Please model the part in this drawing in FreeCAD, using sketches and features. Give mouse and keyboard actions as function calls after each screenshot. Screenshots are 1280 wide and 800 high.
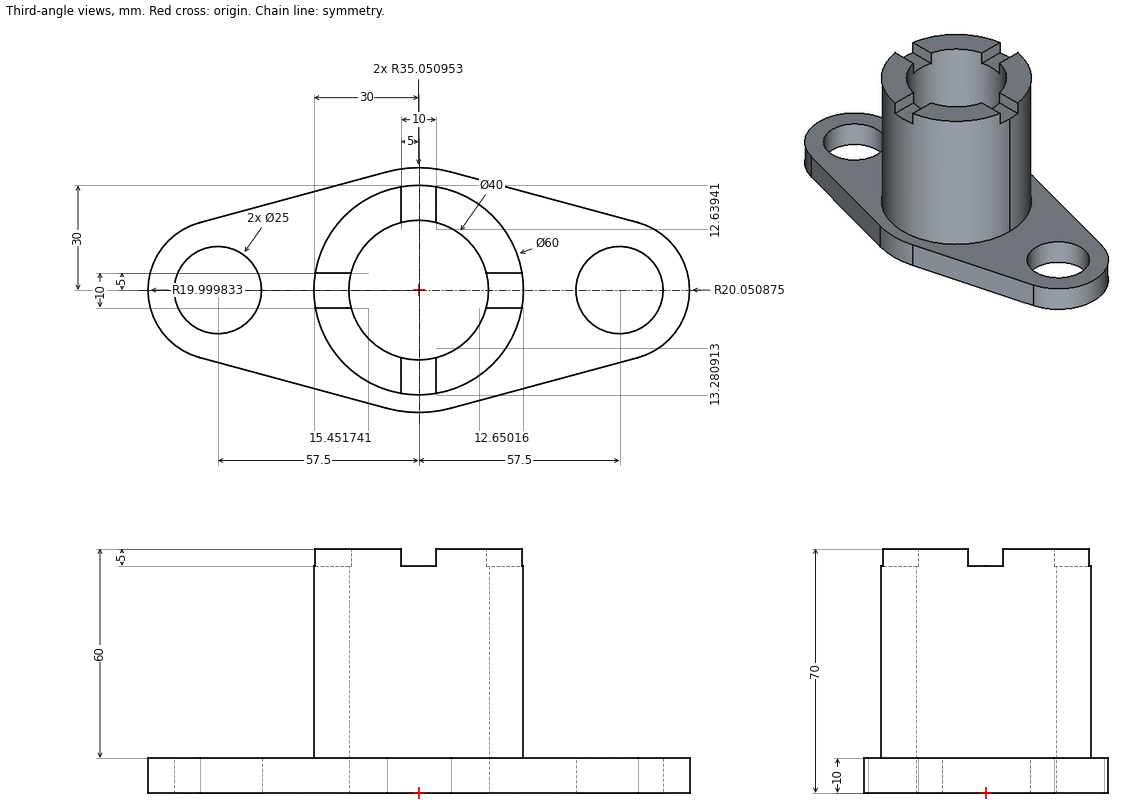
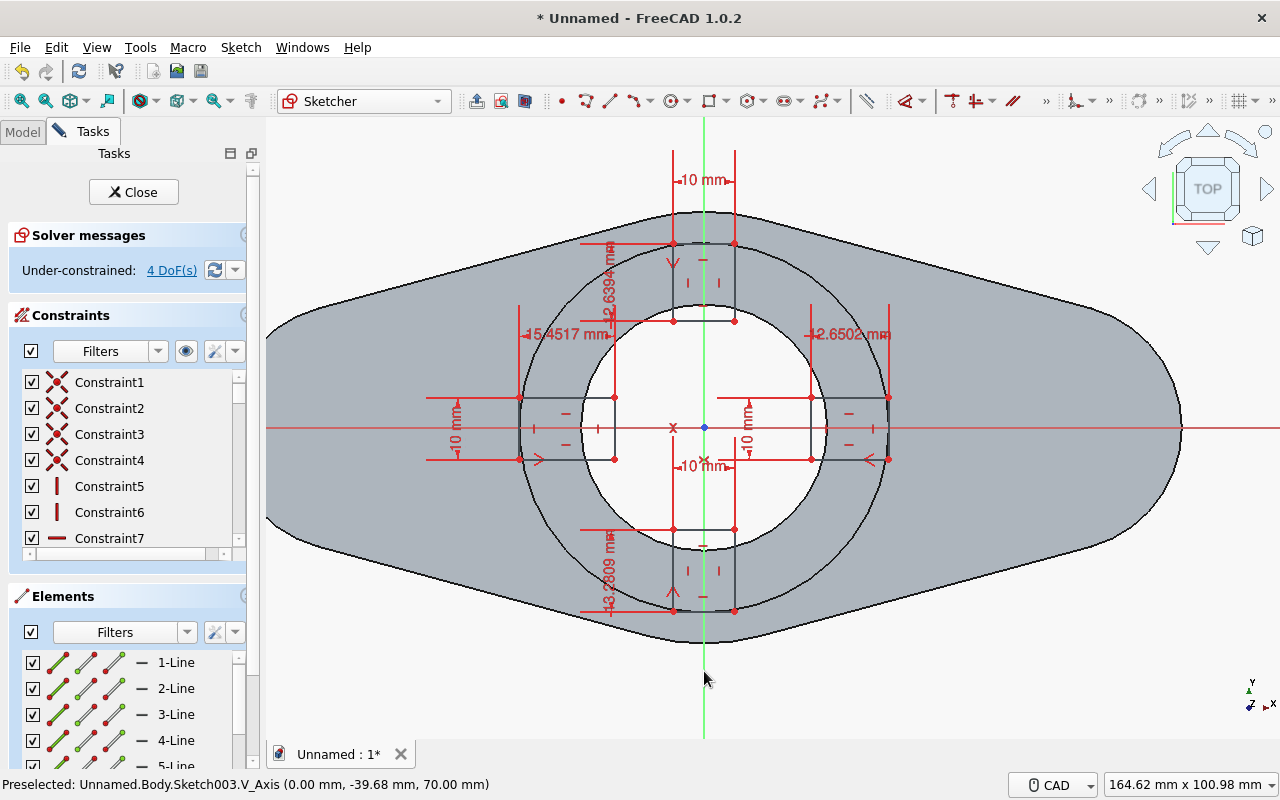
scroll(673, 244, up, 2)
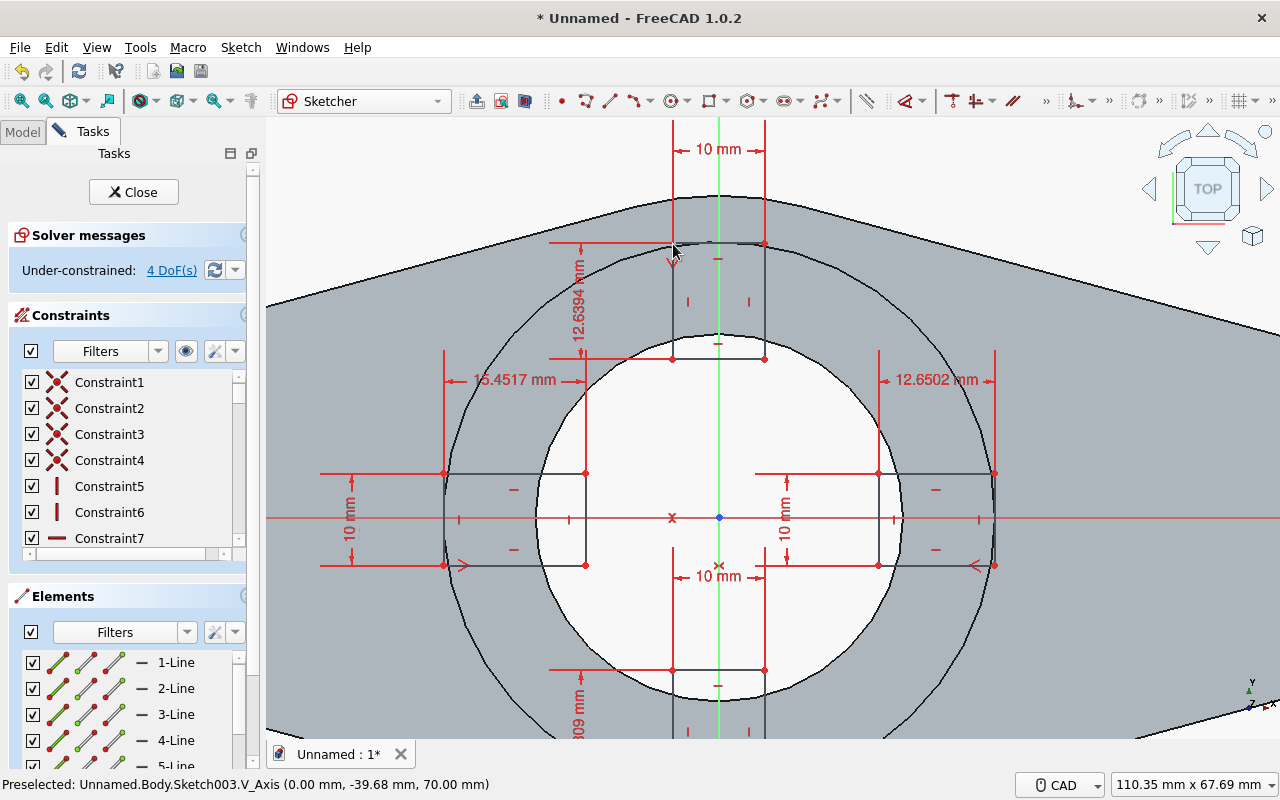
click(673, 243)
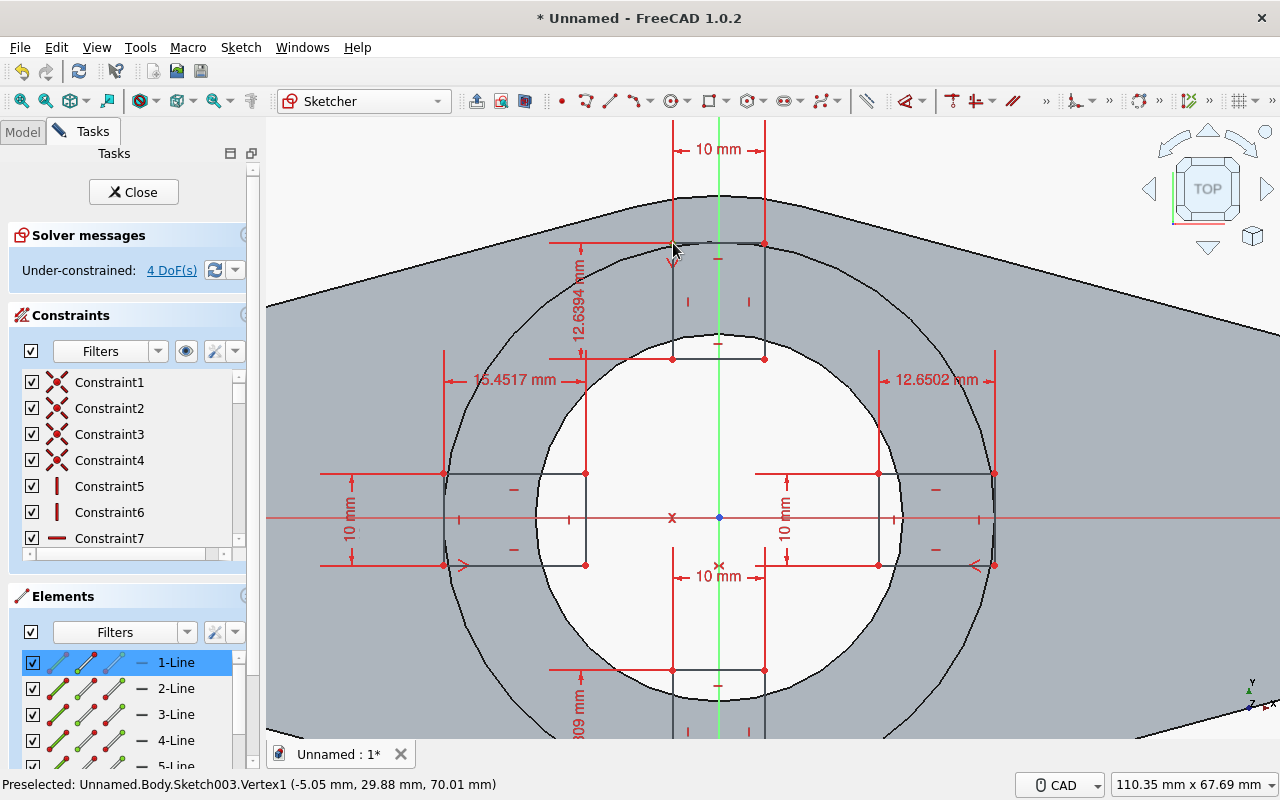
key(l)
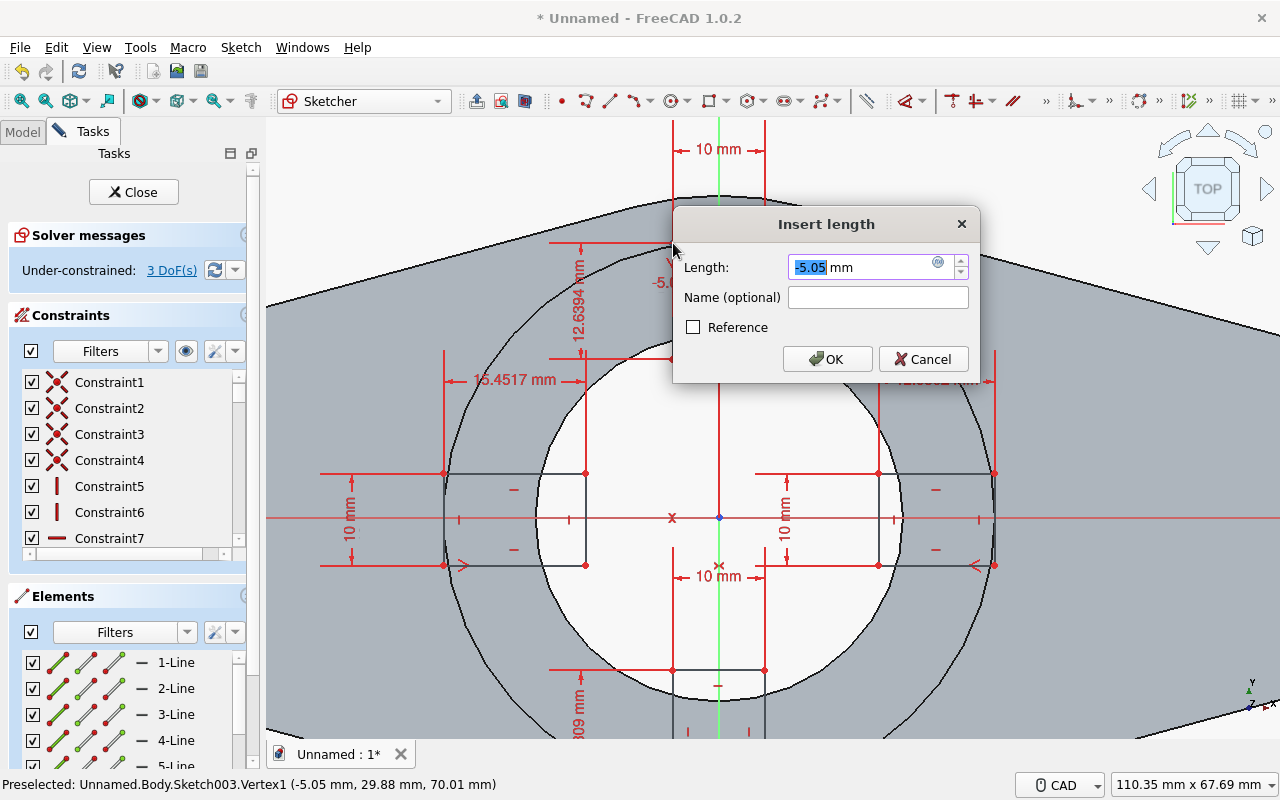
text(-5)
key(Return)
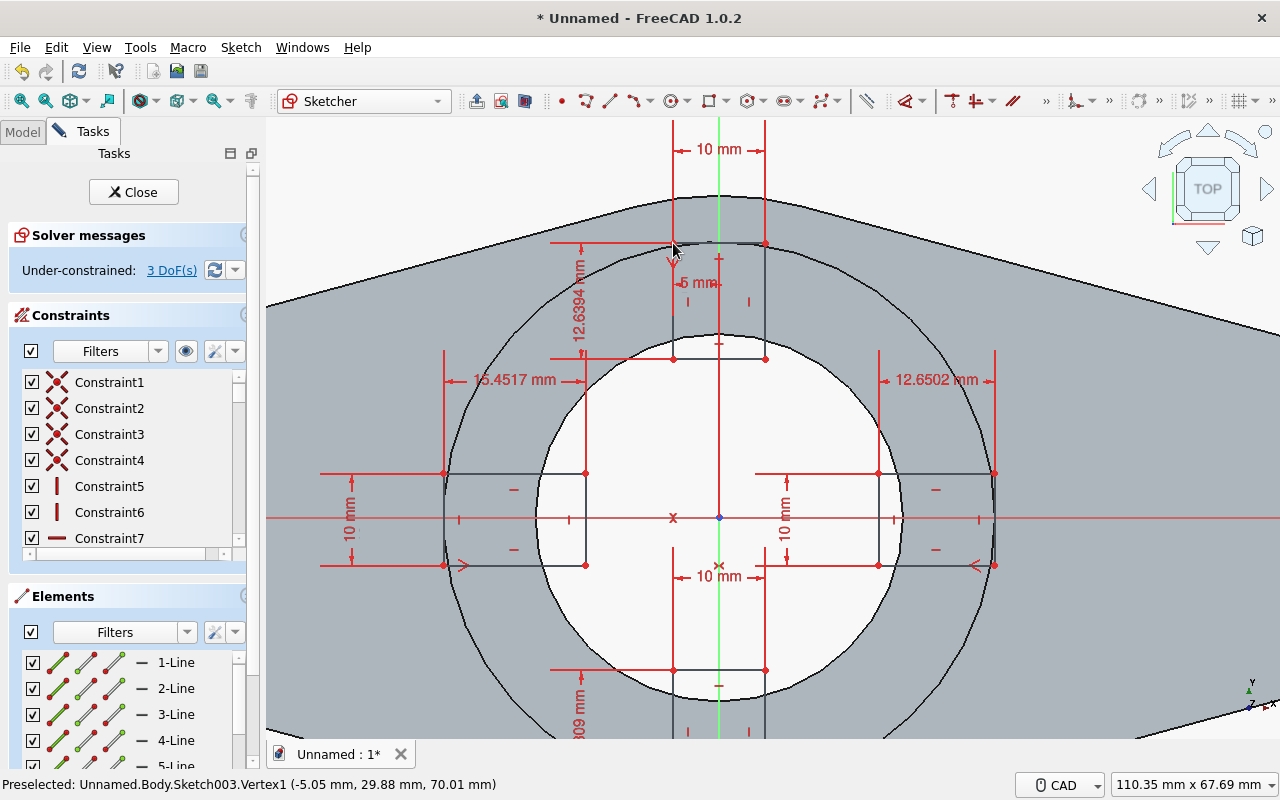
click(444, 474)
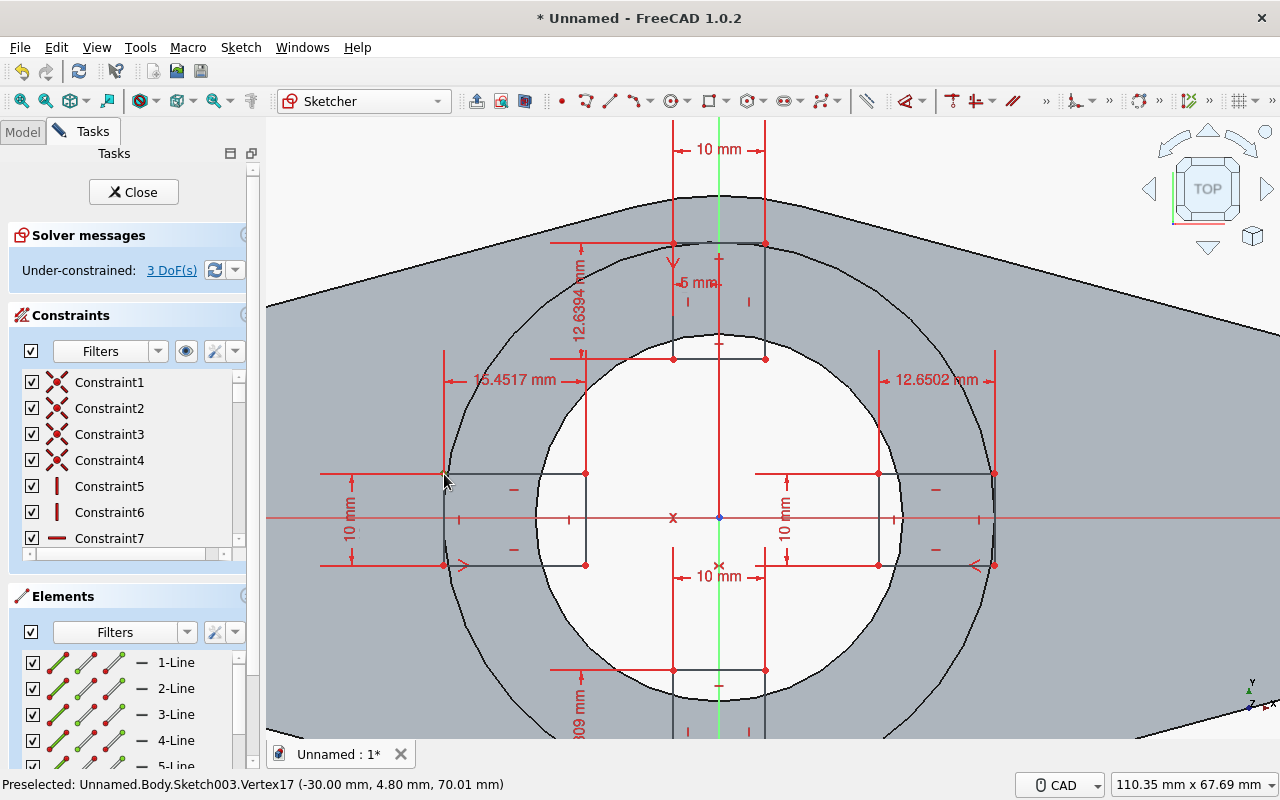
click(924, 102)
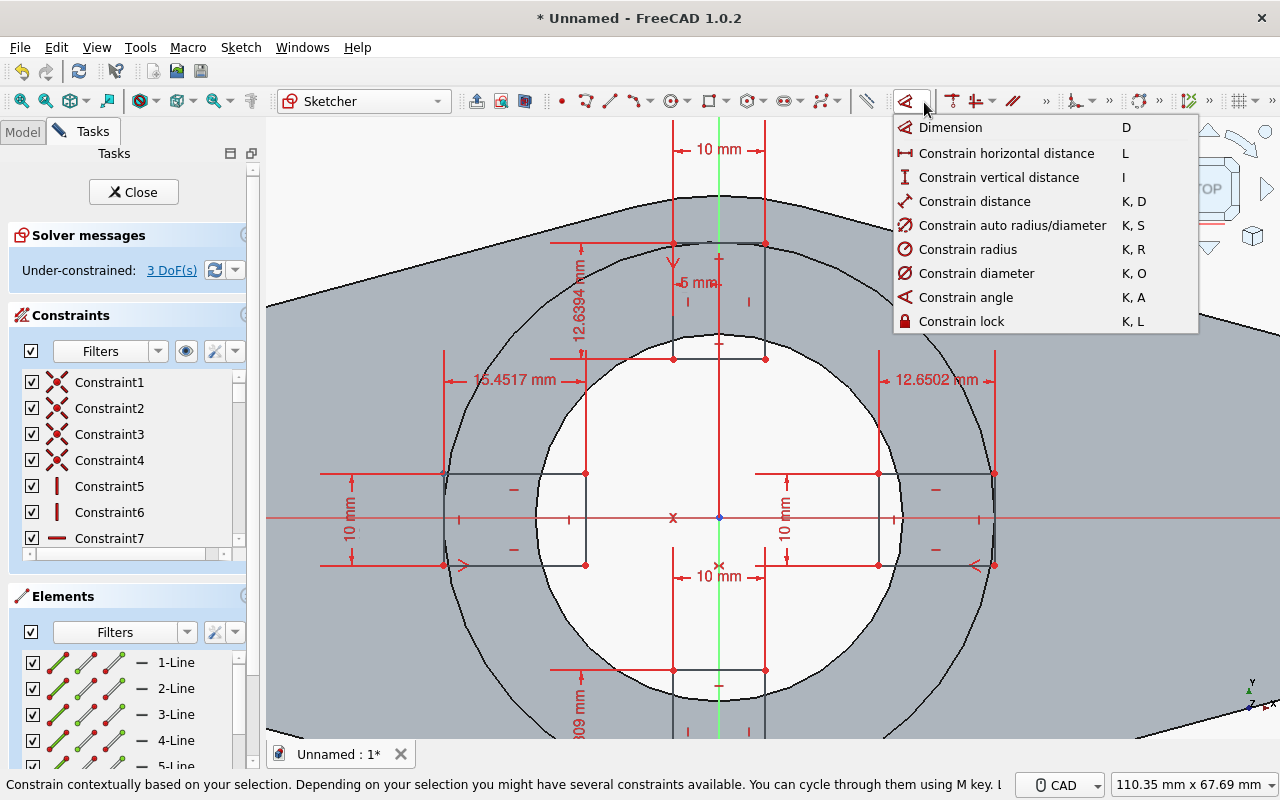
click(1046, 177)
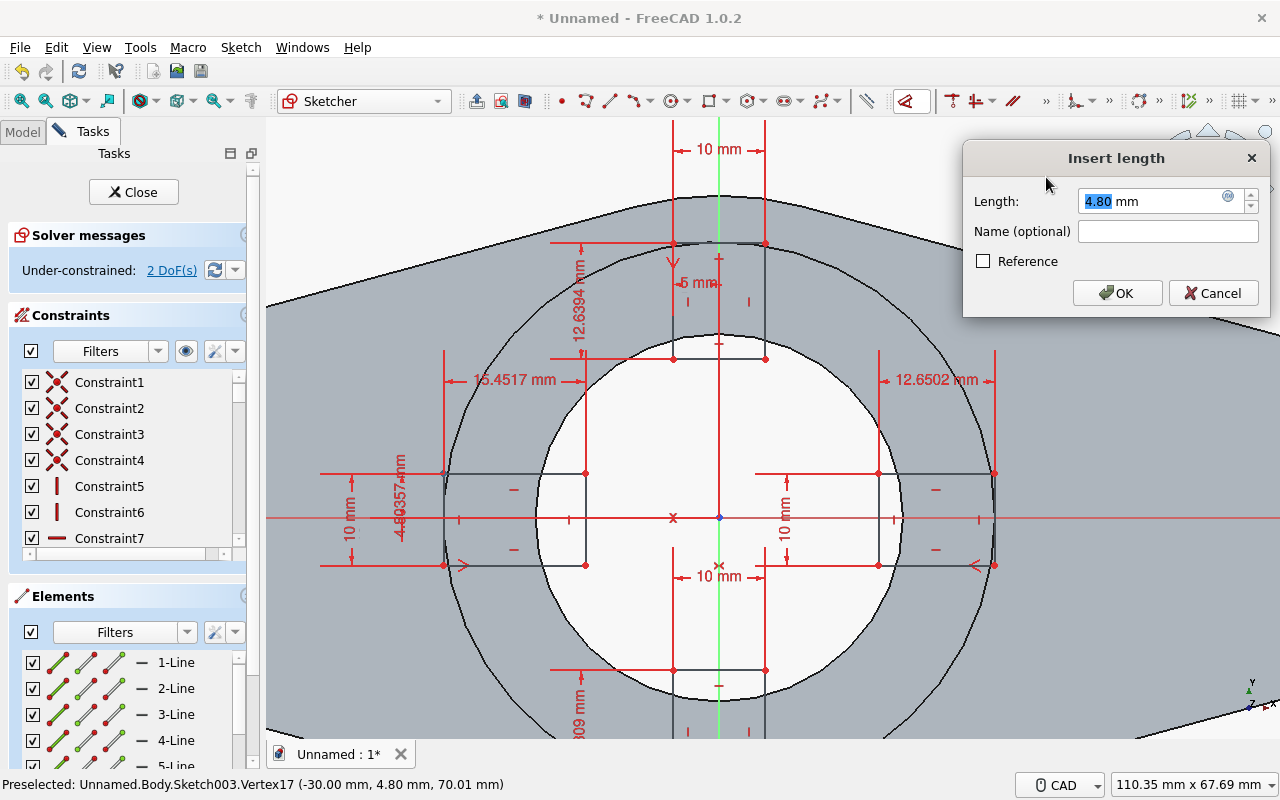
text(5)
key(Return)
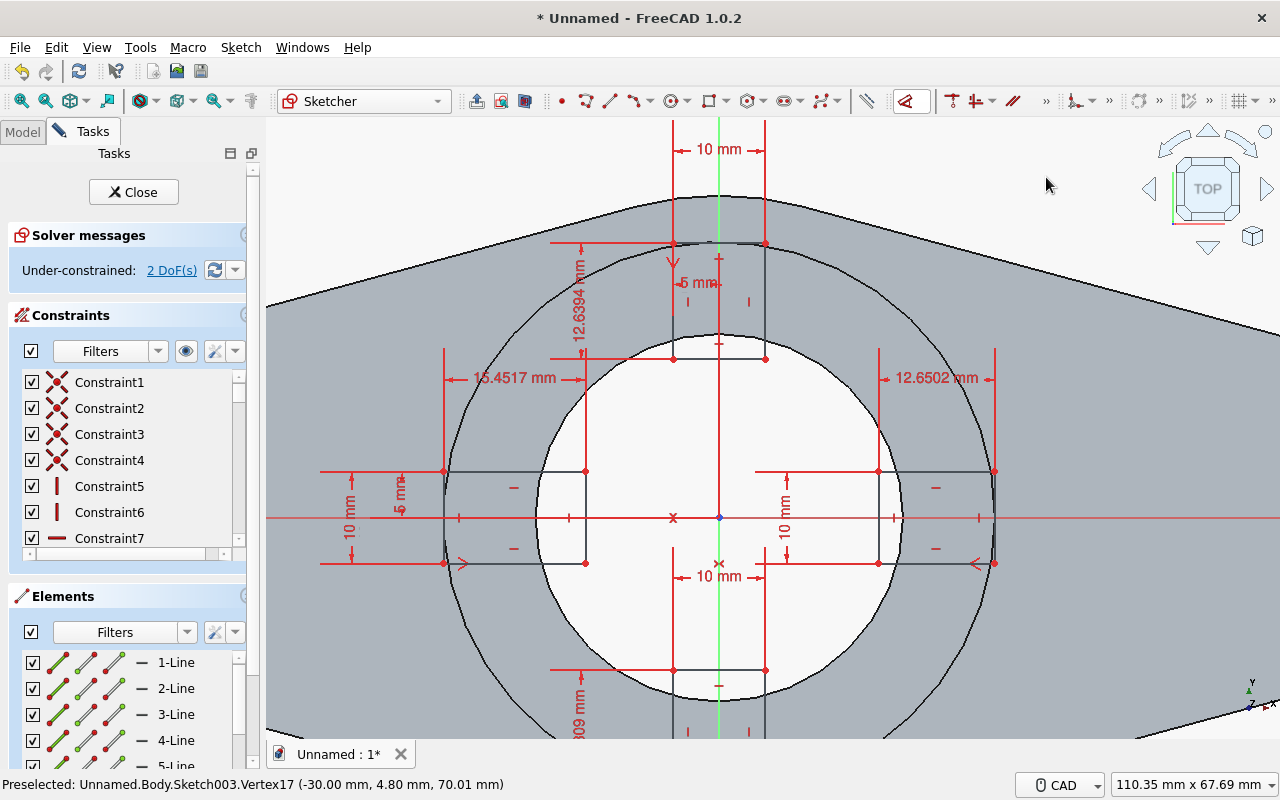
click(673, 243)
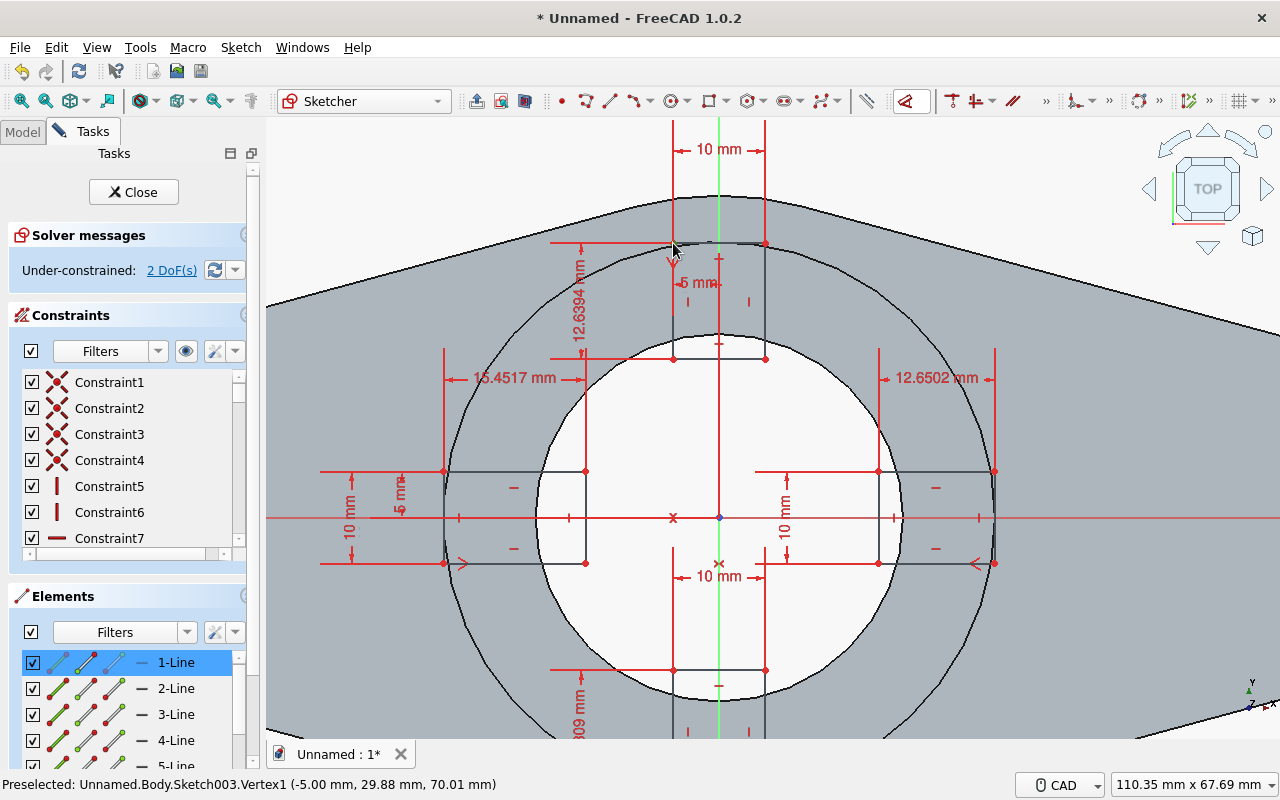
key(i)